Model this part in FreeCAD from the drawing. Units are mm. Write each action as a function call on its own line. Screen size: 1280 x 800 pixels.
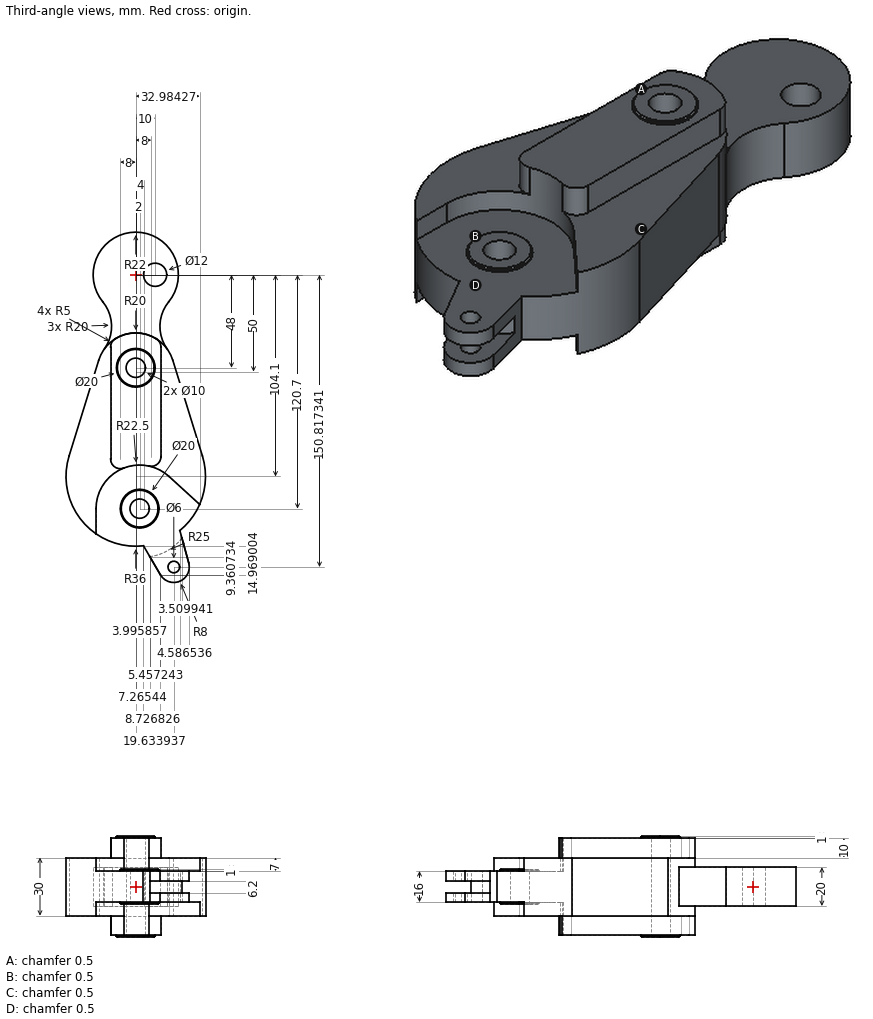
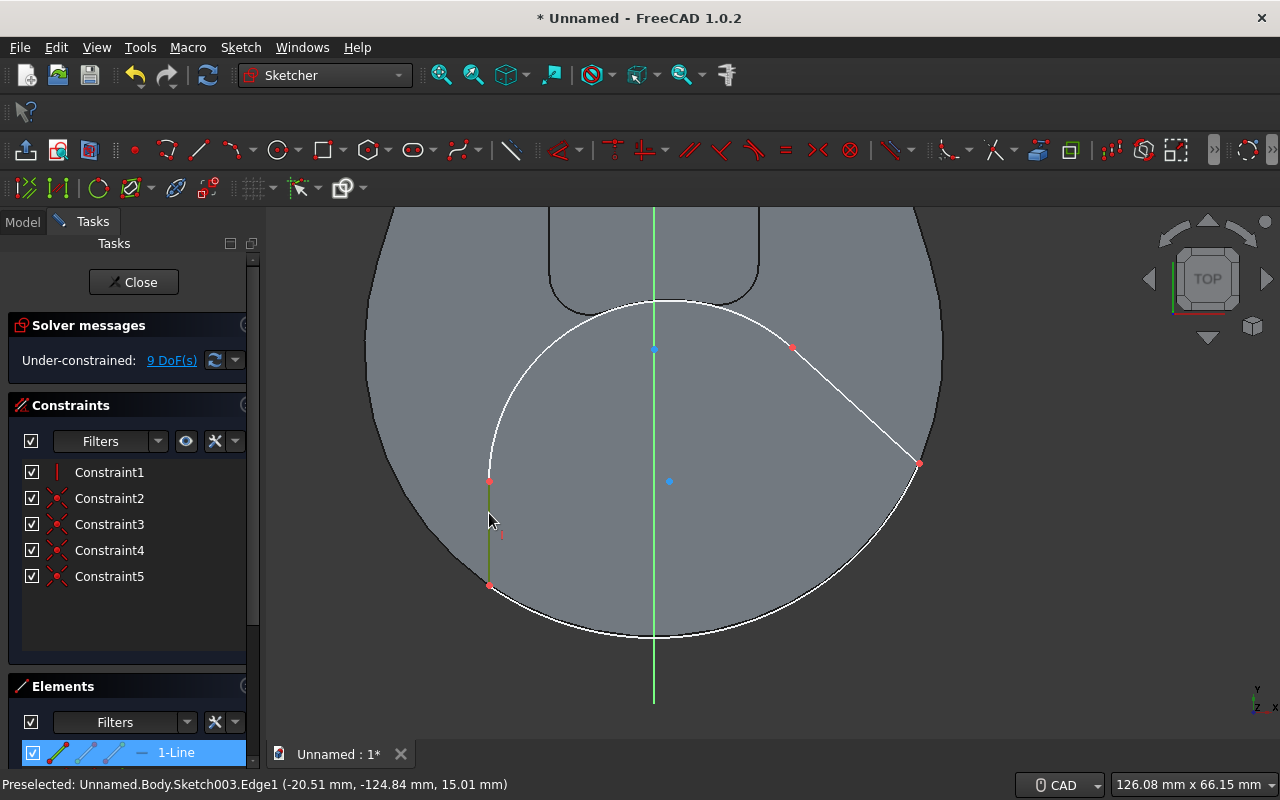
click(678, 301)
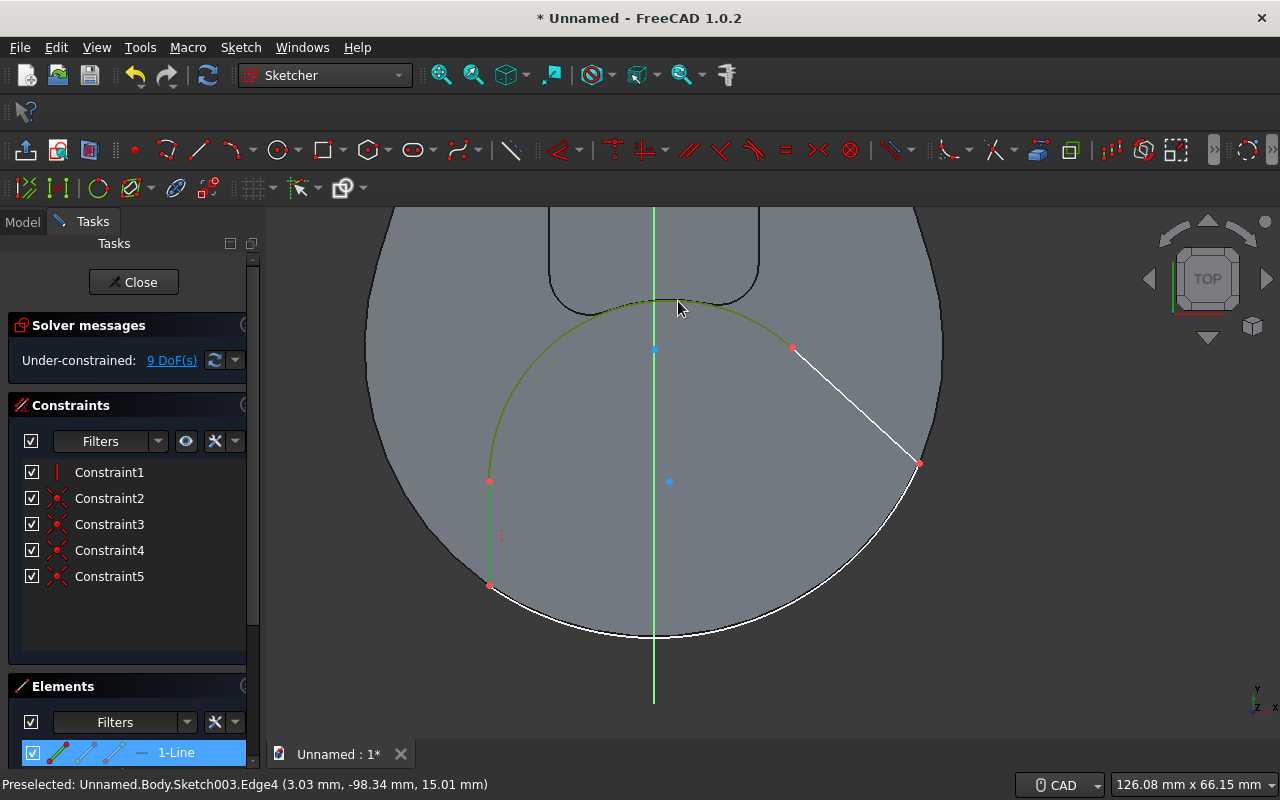
click(754, 150)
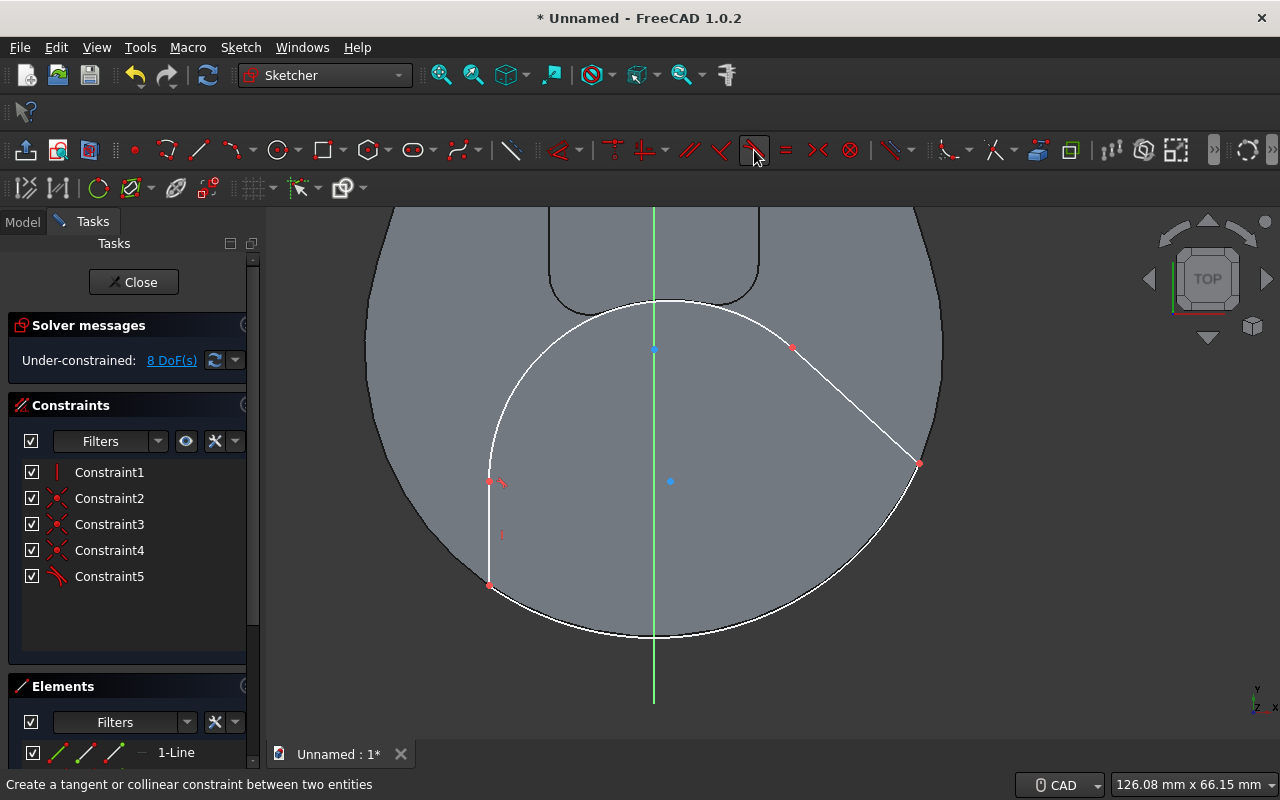
click(881, 429)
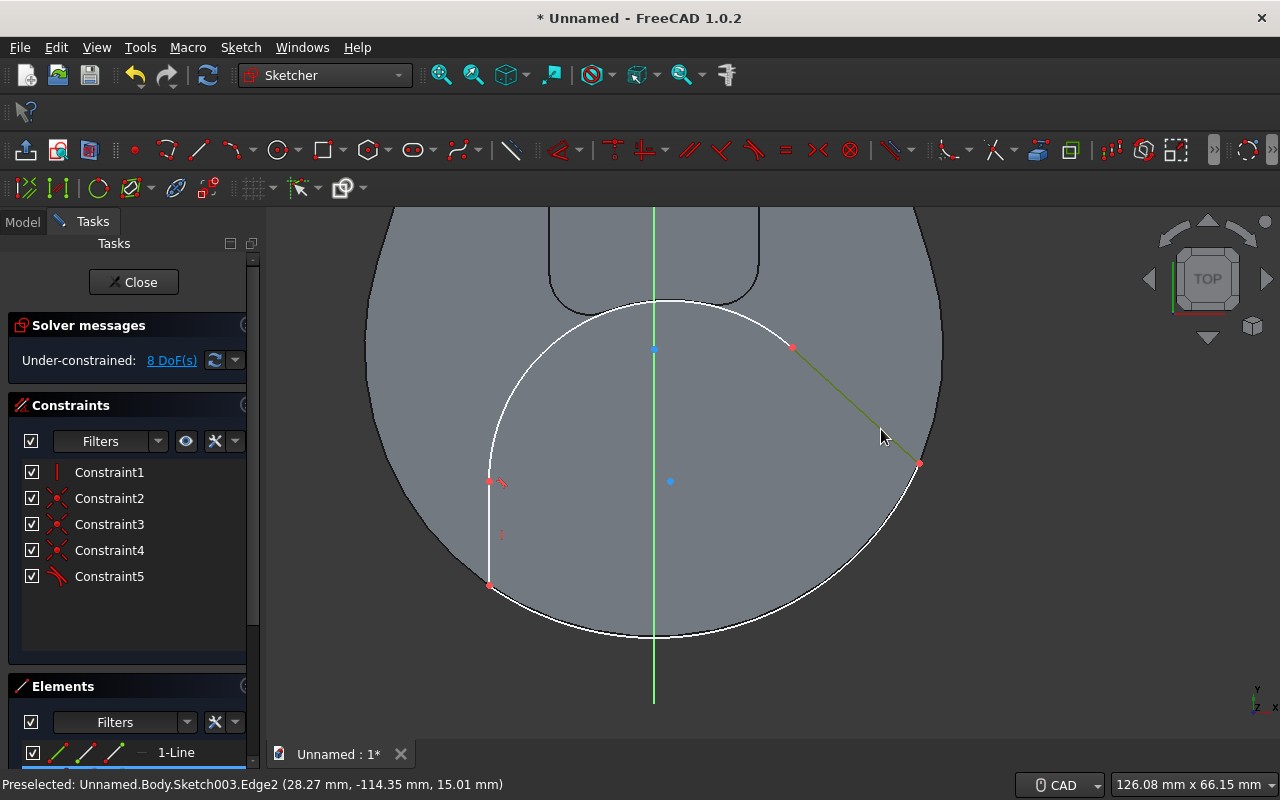
click(678, 301)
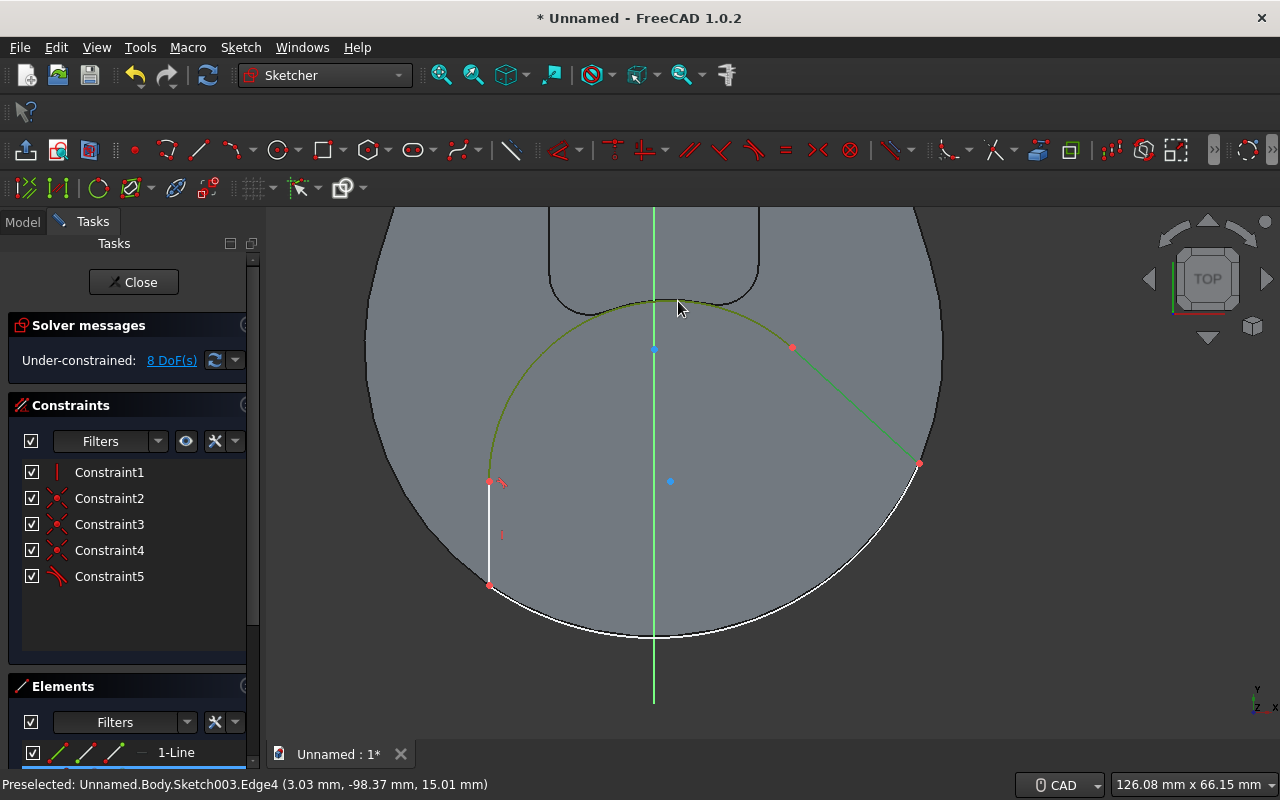
click(754, 150)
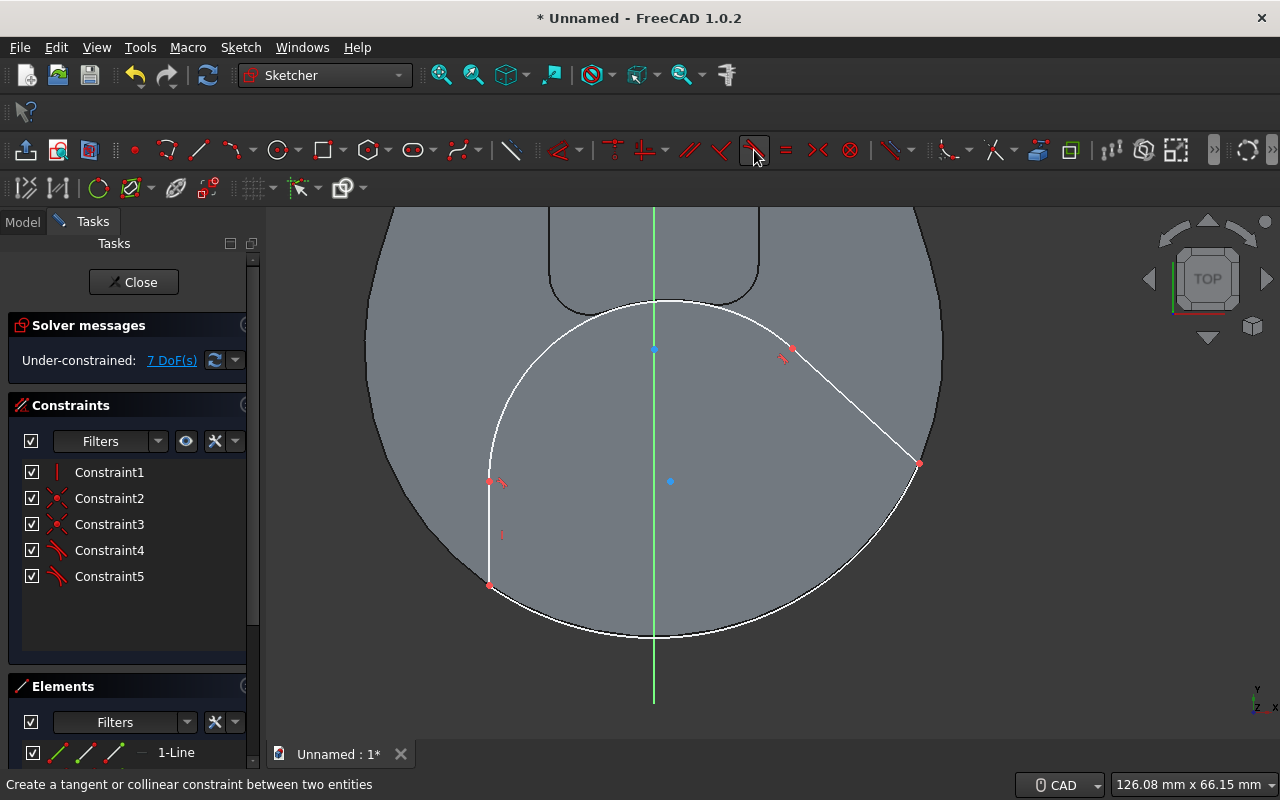
click(654, 349)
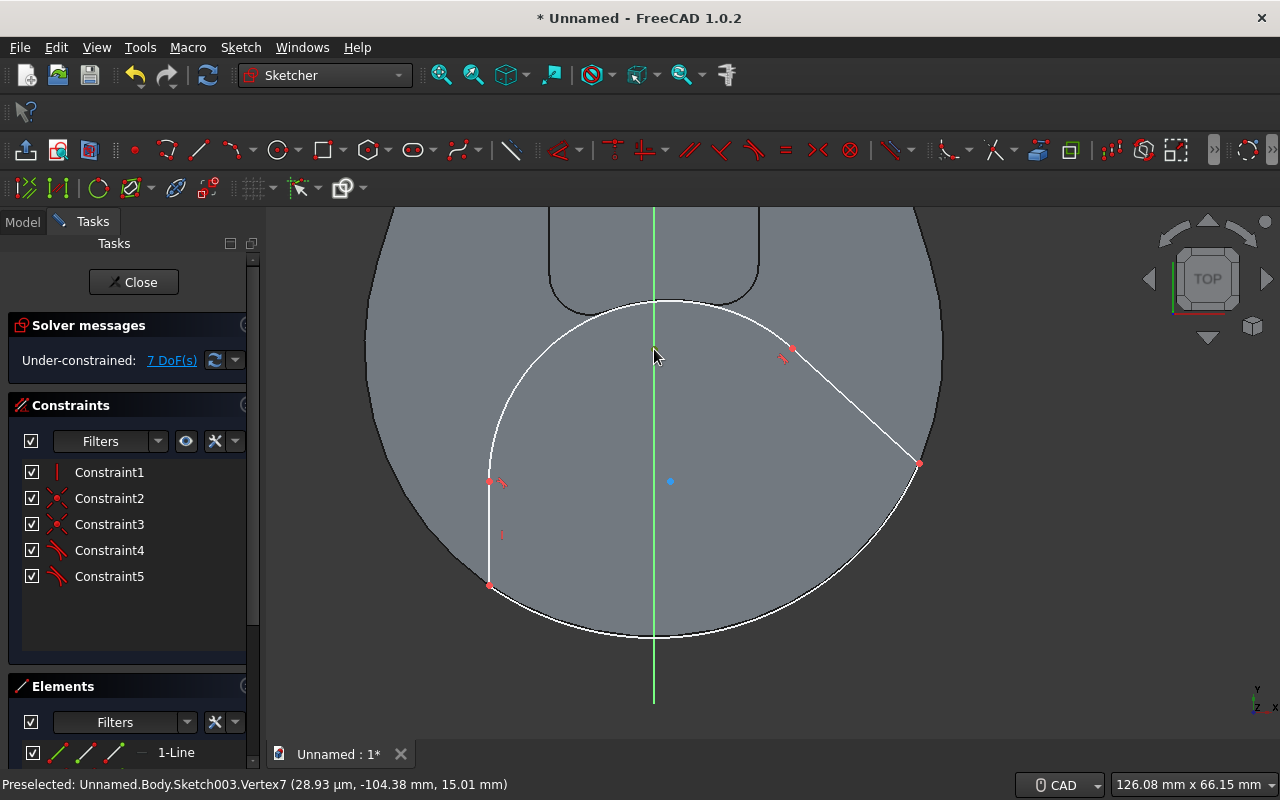
click(654, 677)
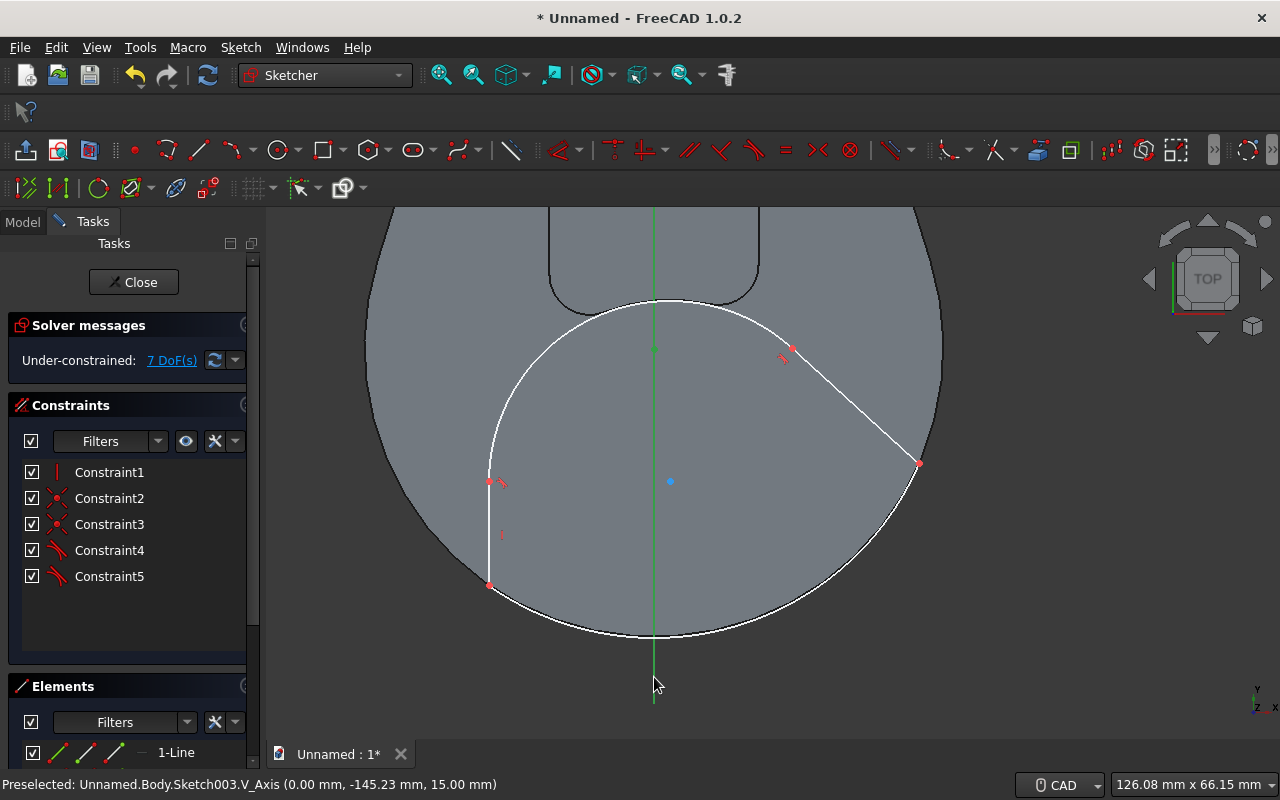
click(614, 150)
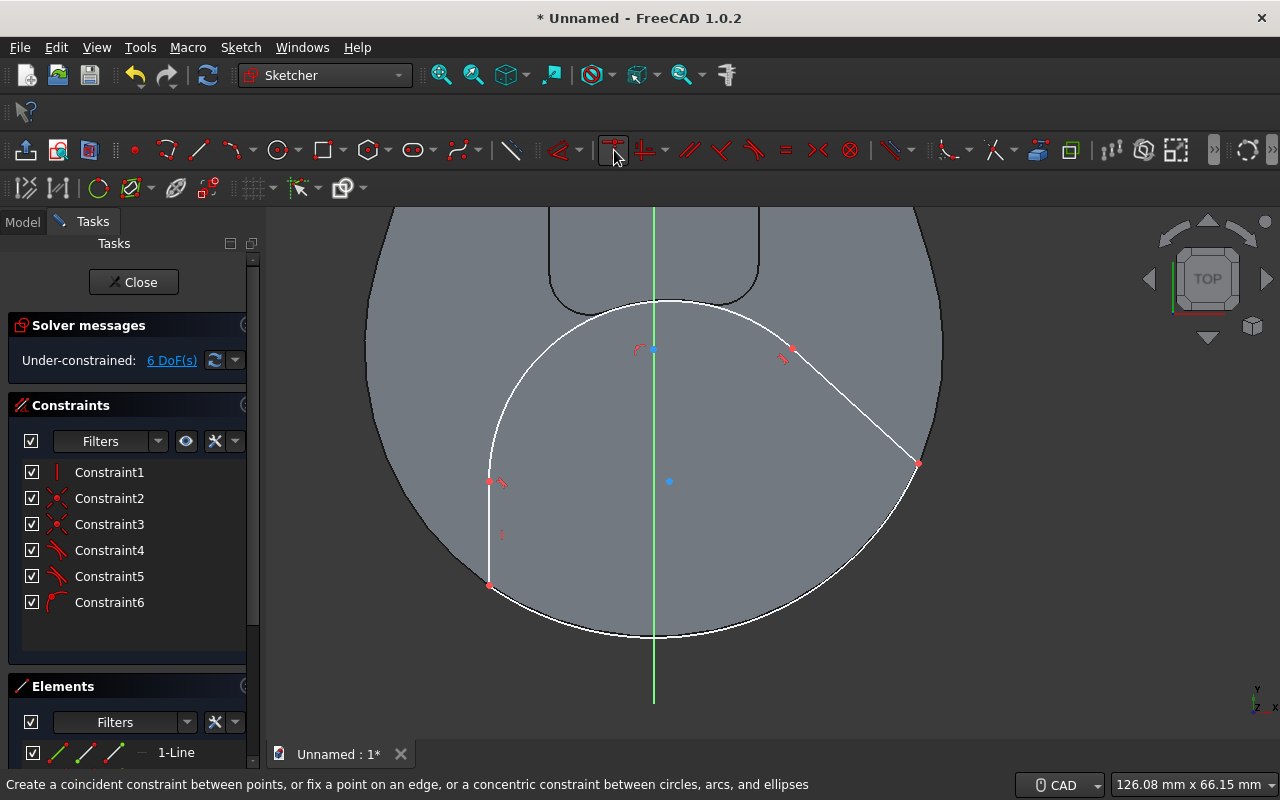
click(558, 150)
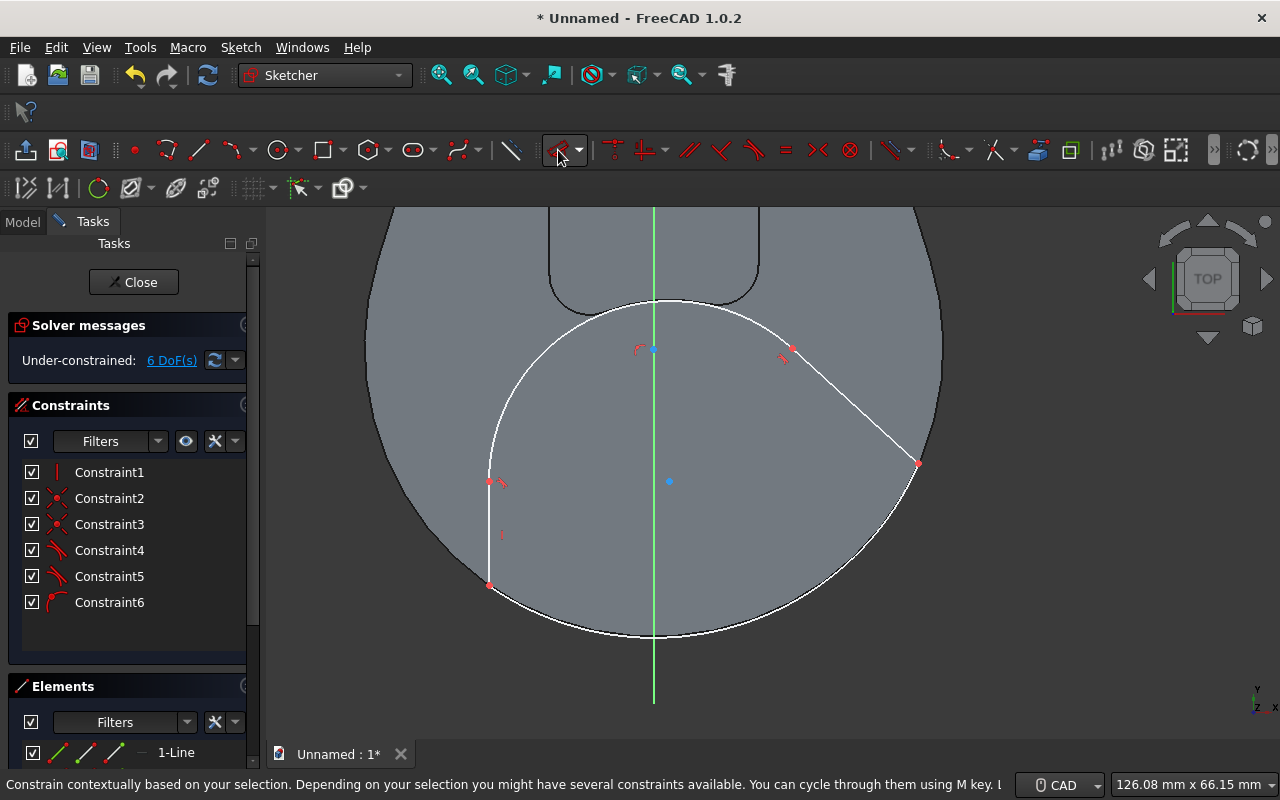
click(632, 637)
click(630, 669)